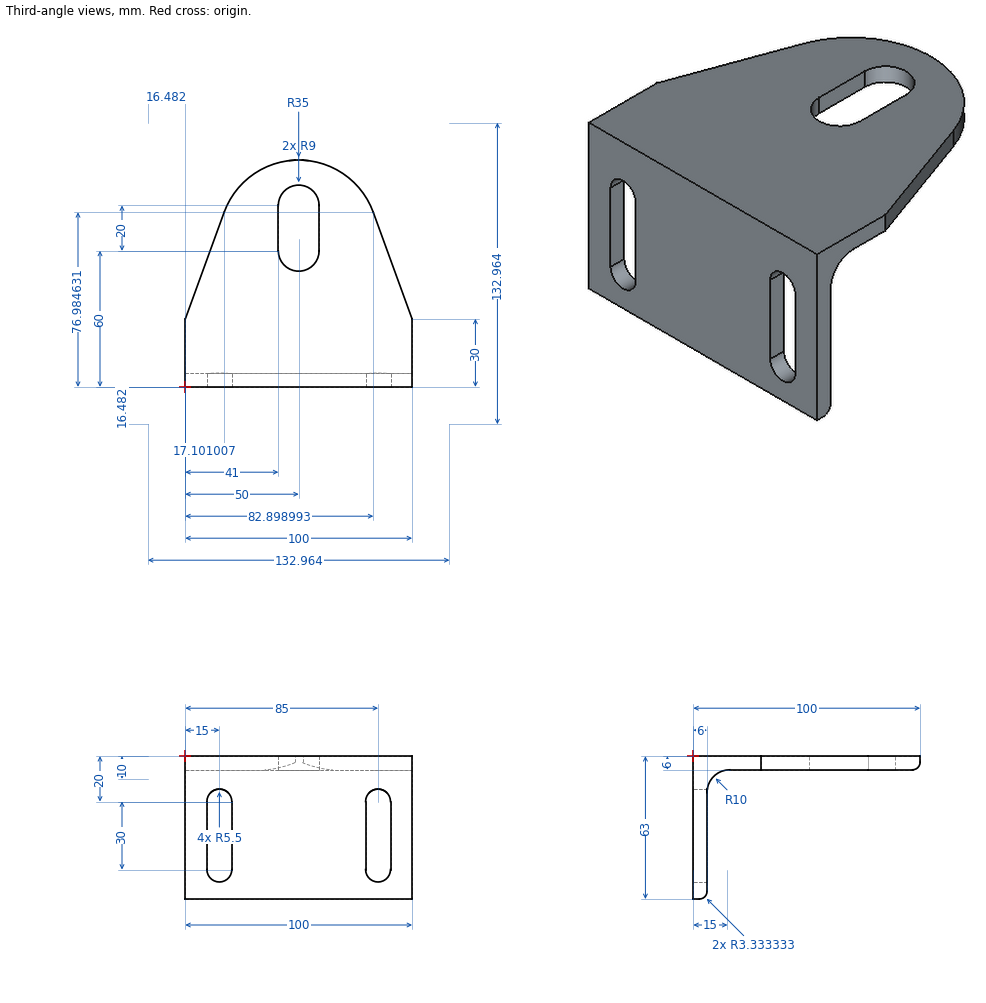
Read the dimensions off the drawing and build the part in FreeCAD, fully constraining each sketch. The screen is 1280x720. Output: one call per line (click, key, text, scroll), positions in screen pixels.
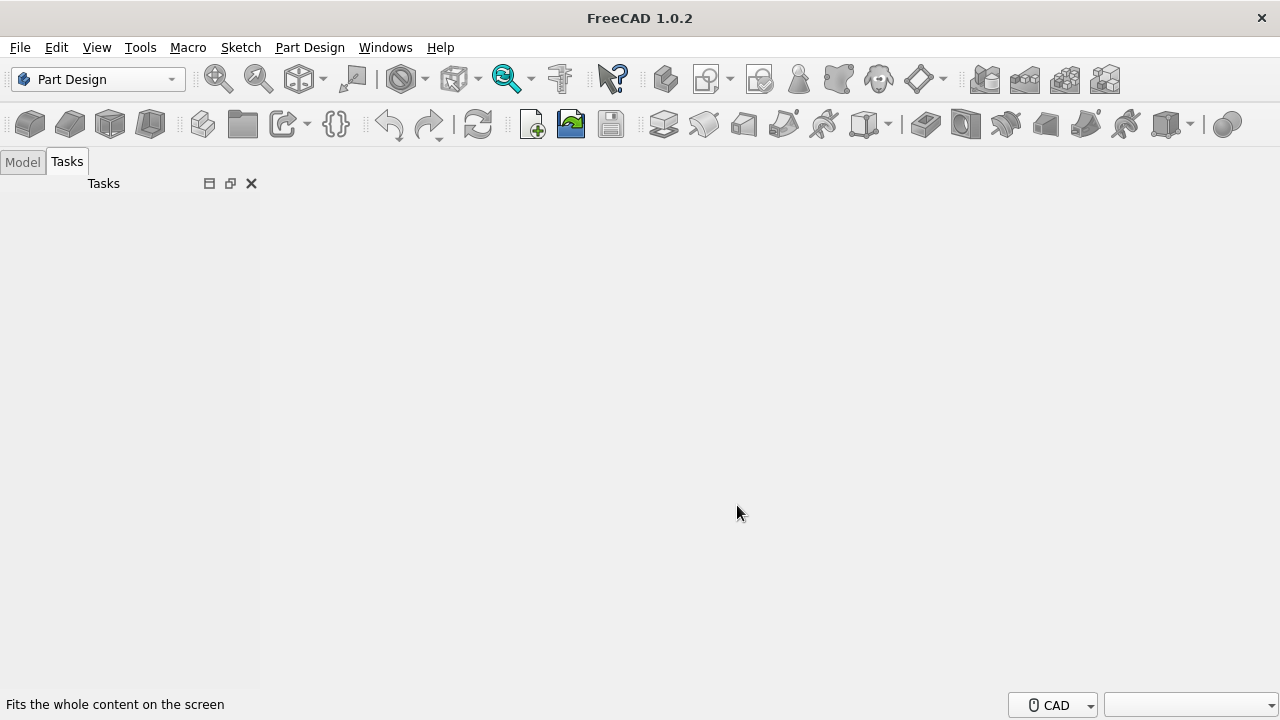
click(532, 124)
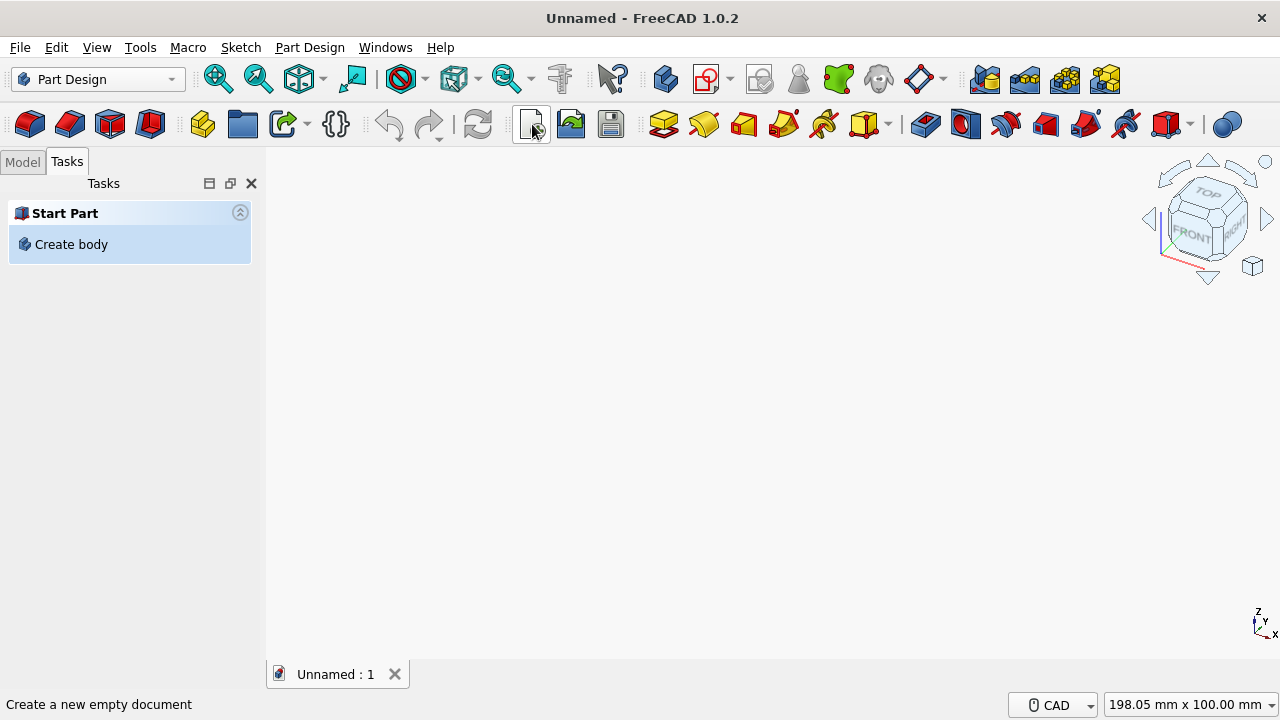
click(706, 80)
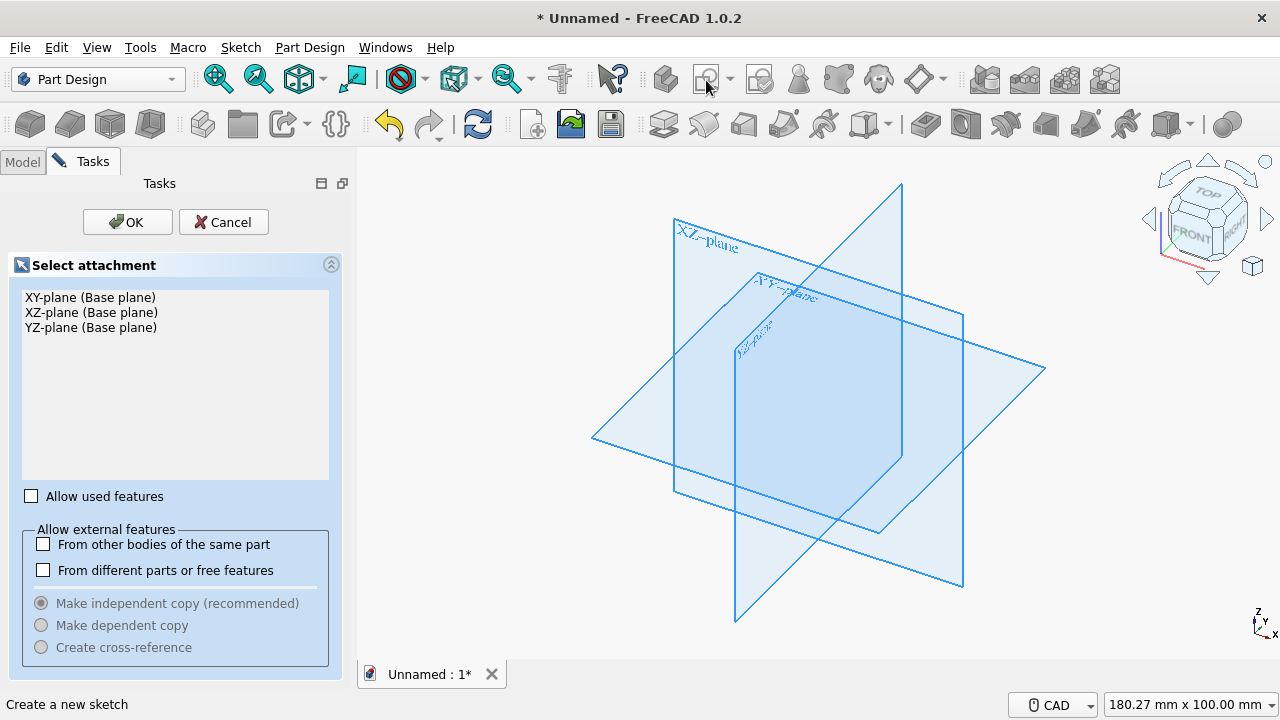
click(82, 328)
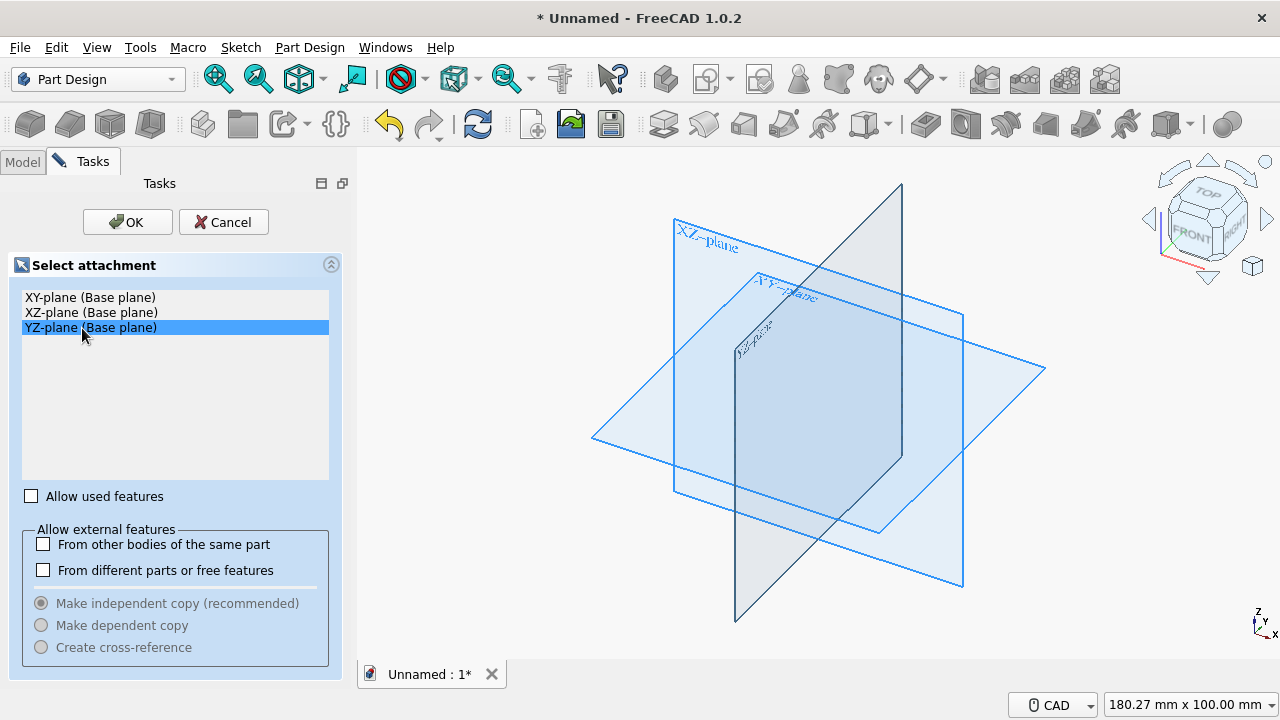
click(128, 222)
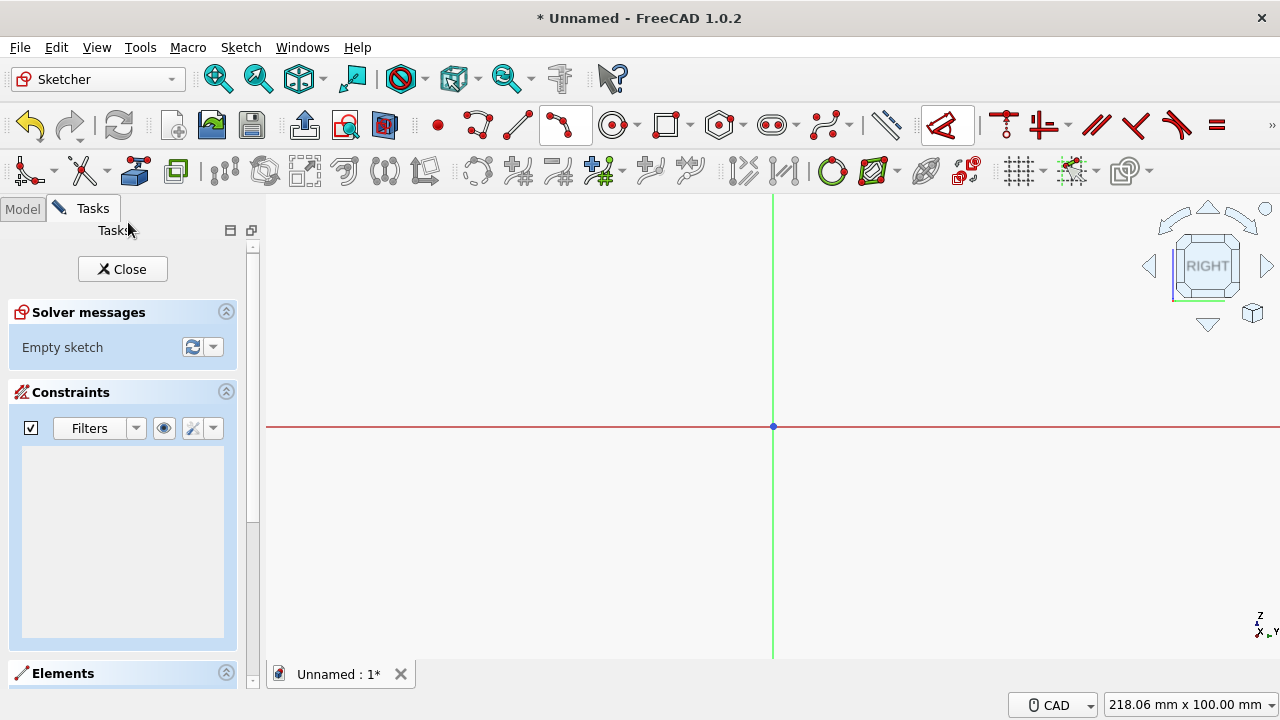
scroll(294, 222, down, 2)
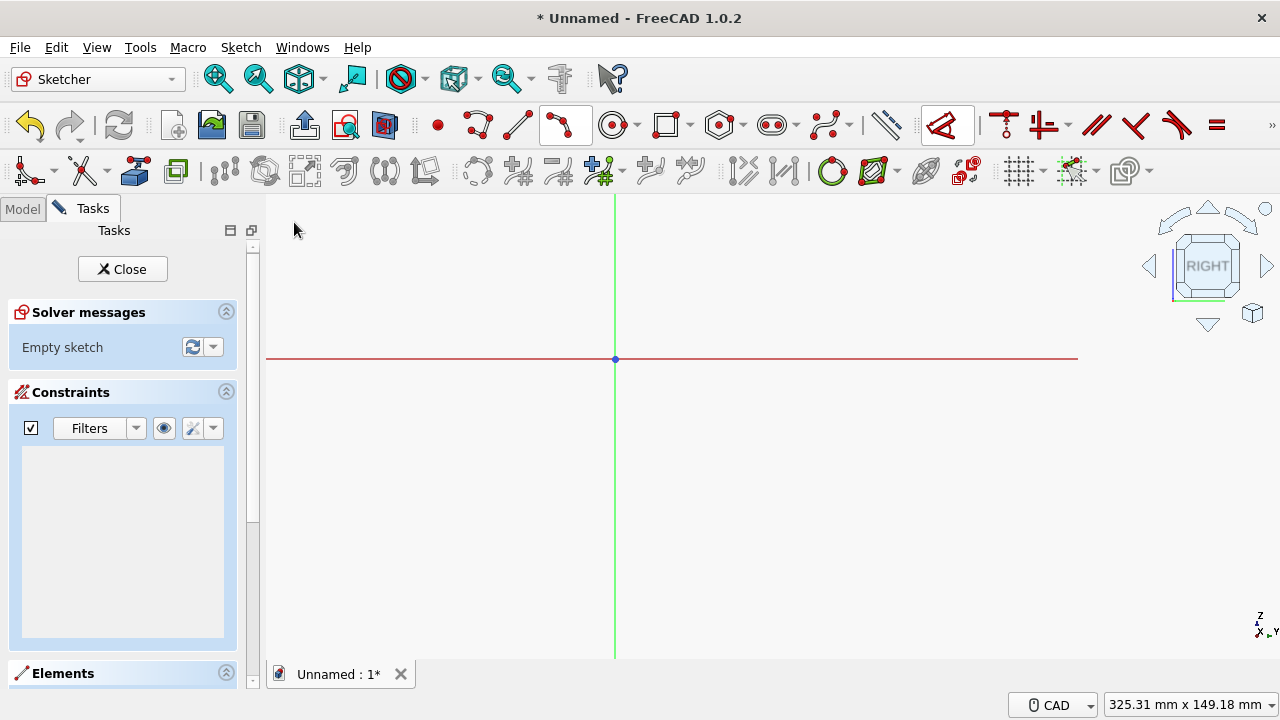
scroll(906, 520, up, 2)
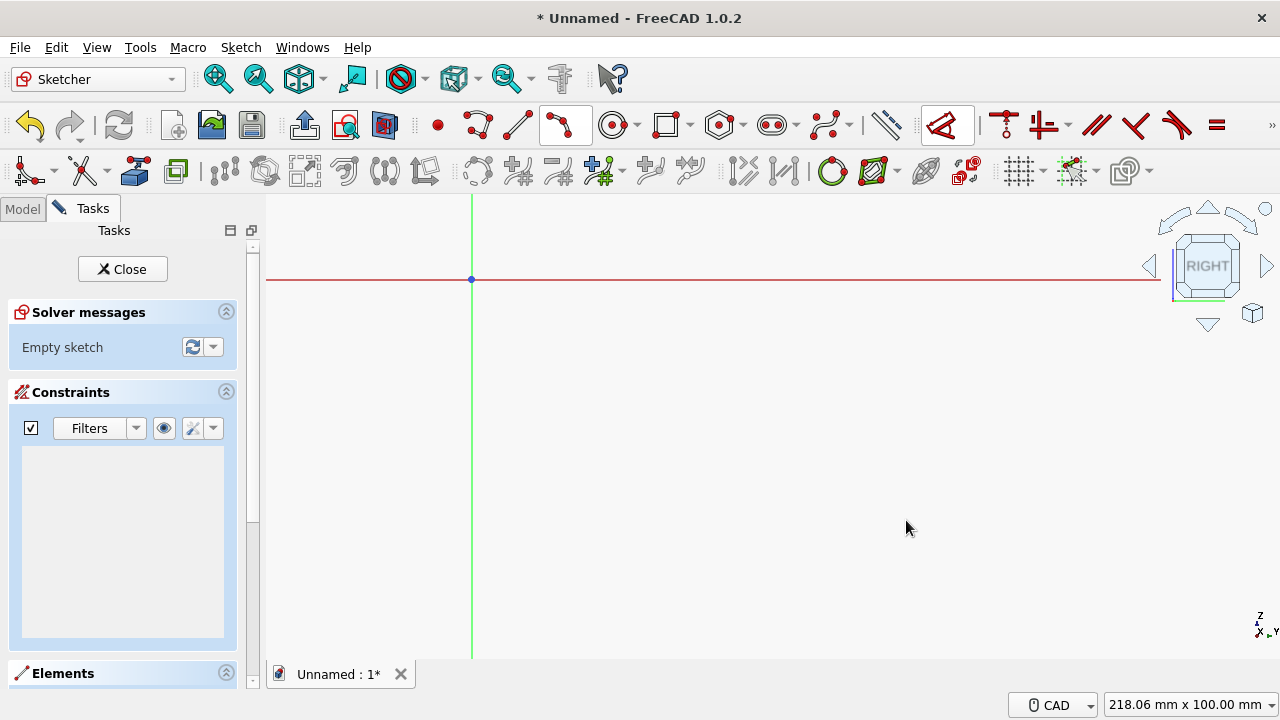
click(518, 126)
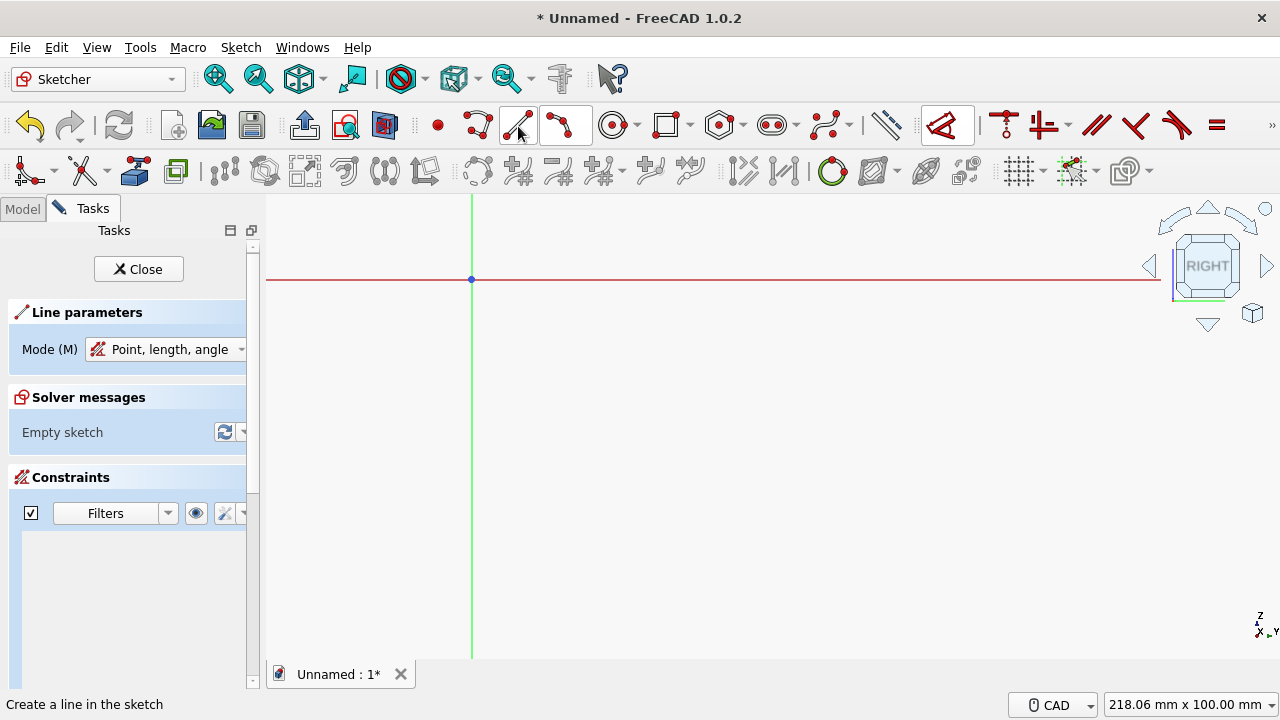
click(500, 557)
click(500, 354)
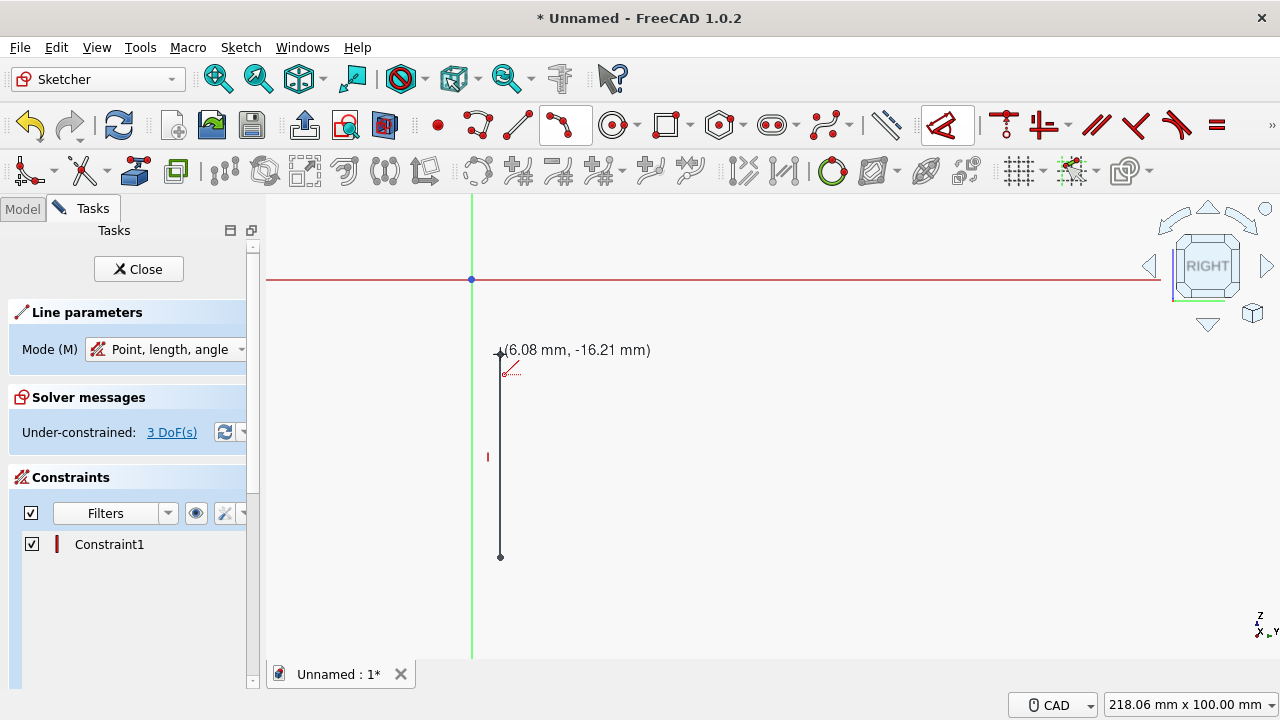
click(546, 308)
click(921, 308)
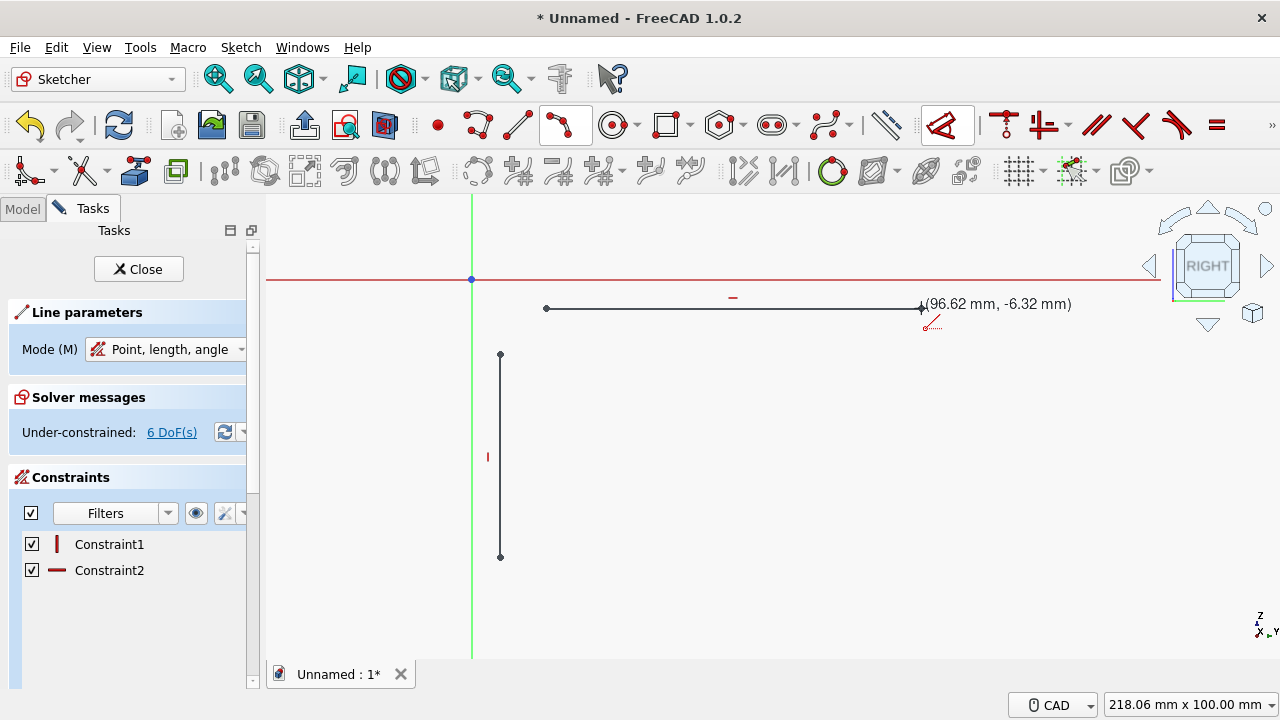
click(478, 126)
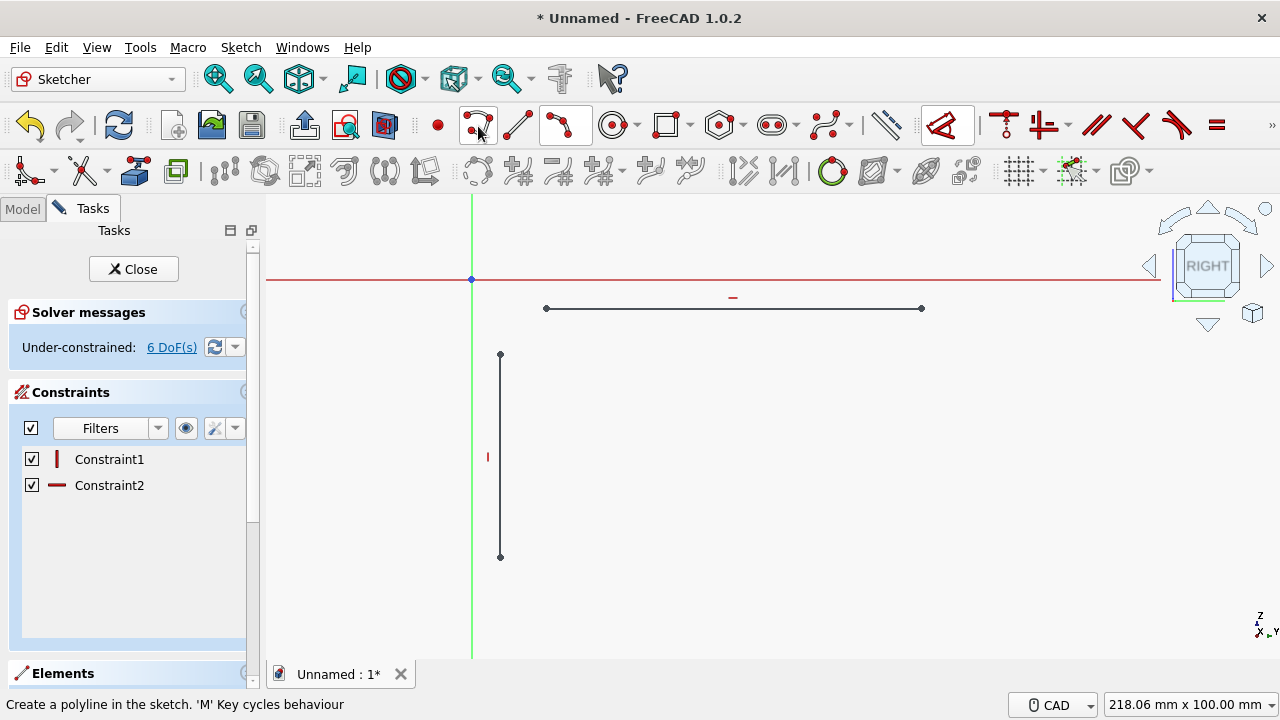
scroll(937, 292, up, 2)